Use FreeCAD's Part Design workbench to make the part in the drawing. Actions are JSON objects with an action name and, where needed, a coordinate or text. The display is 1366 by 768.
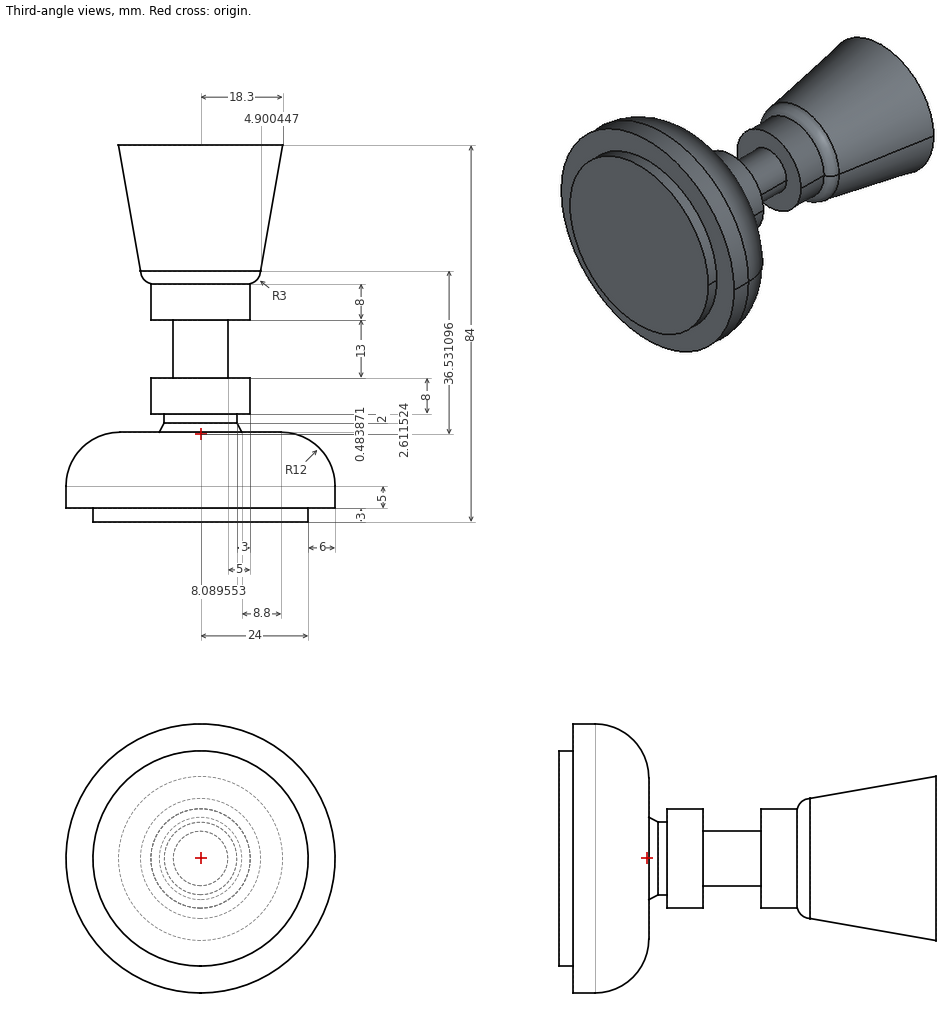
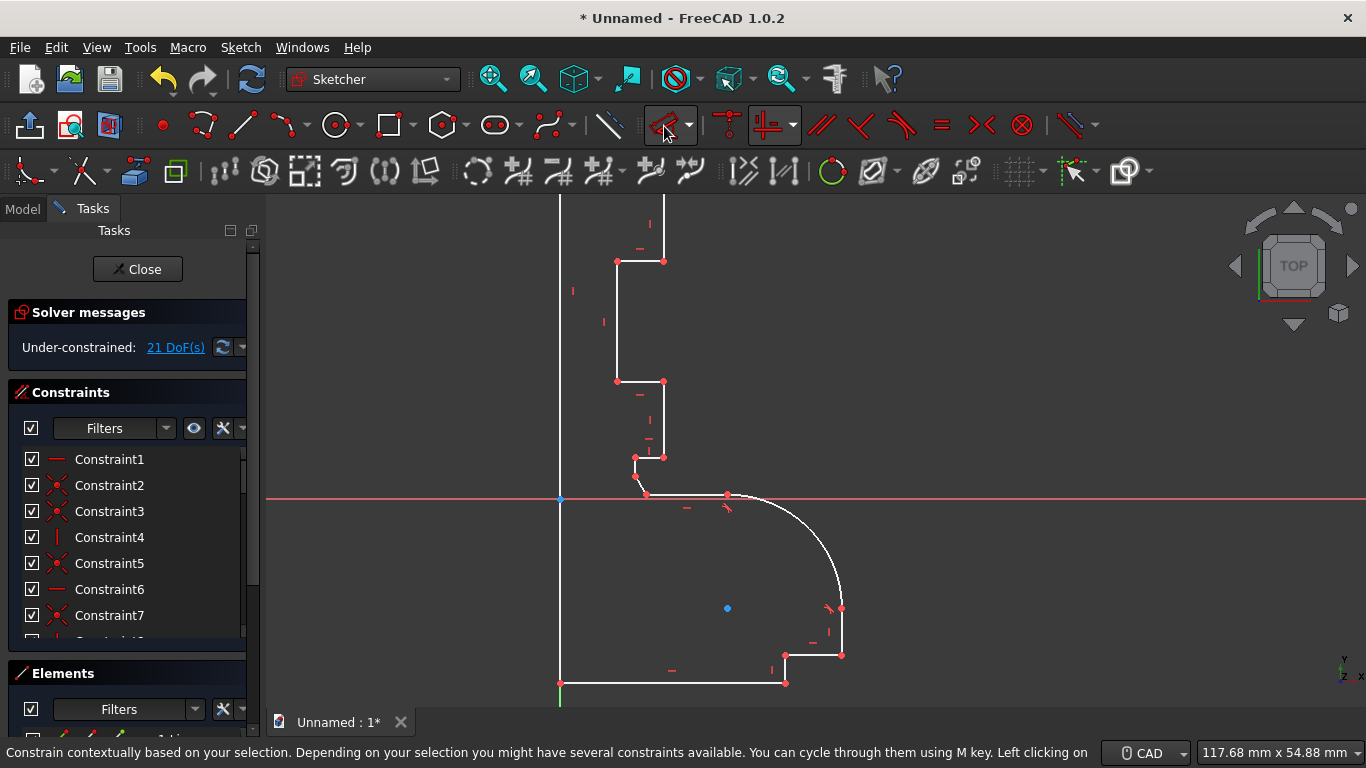
{"action": "scroll", "coordinate": [786, 582], "scroll_direction": "down", "scroll_amount": 4}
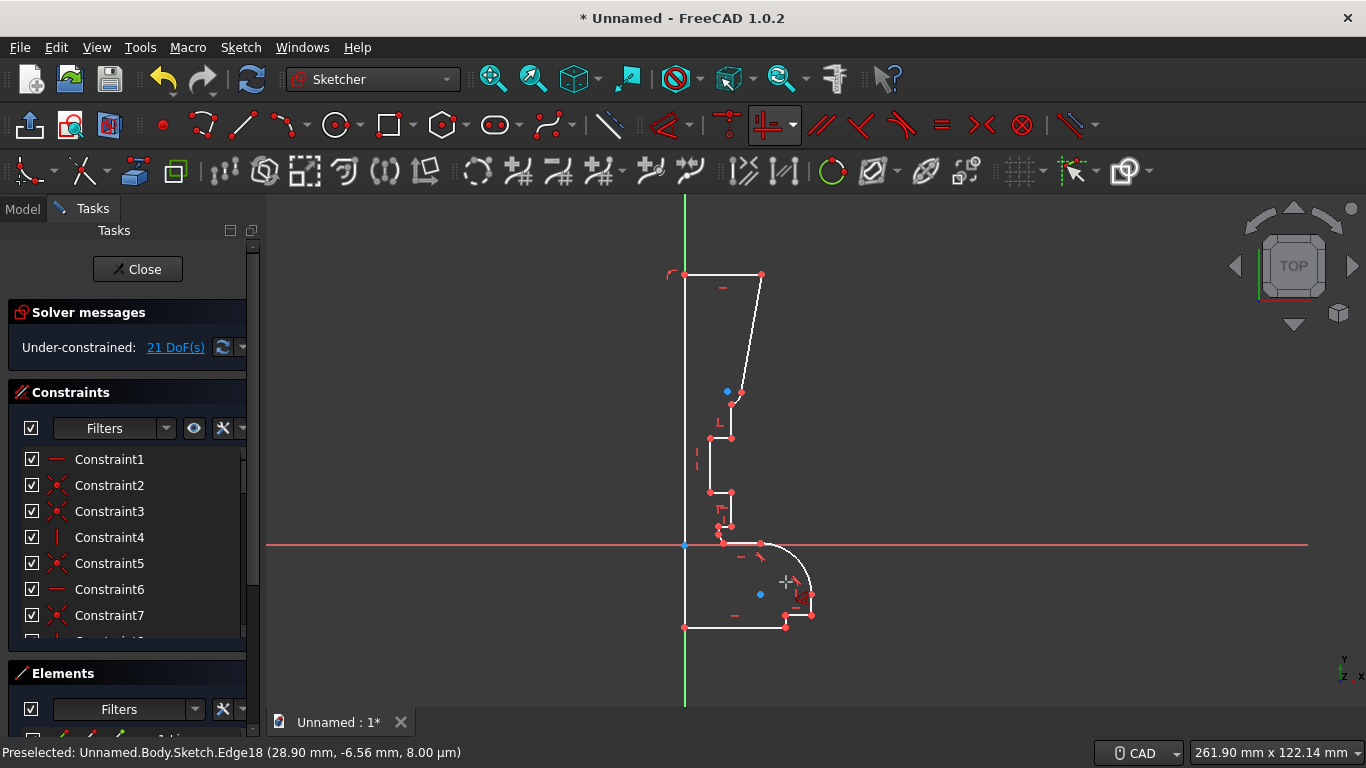
{"action": "scroll", "coordinate": [736, 402], "scroll_direction": "up", "scroll_amount": 6}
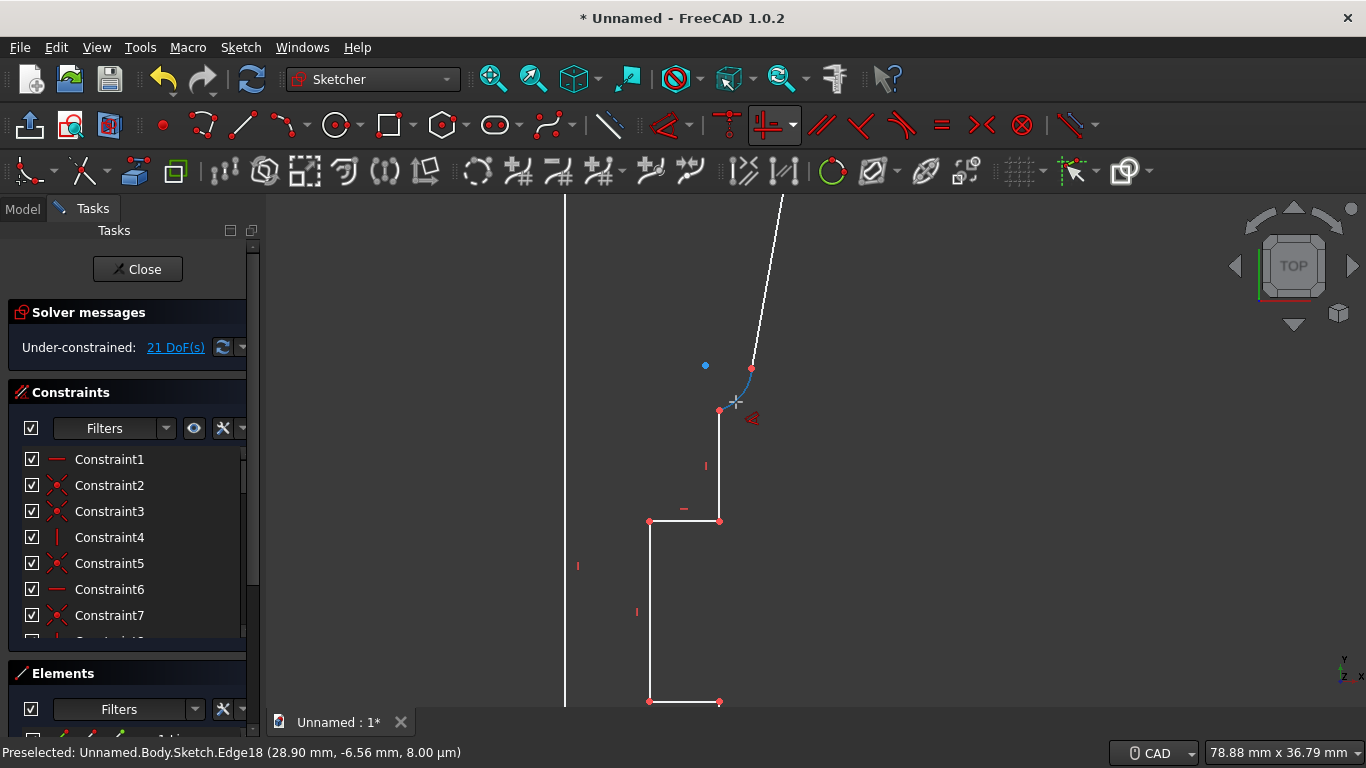
{"action": "left_click", "coordinate": [734, 402]}
{"action": "left_click", "coordinate": [754, 427]}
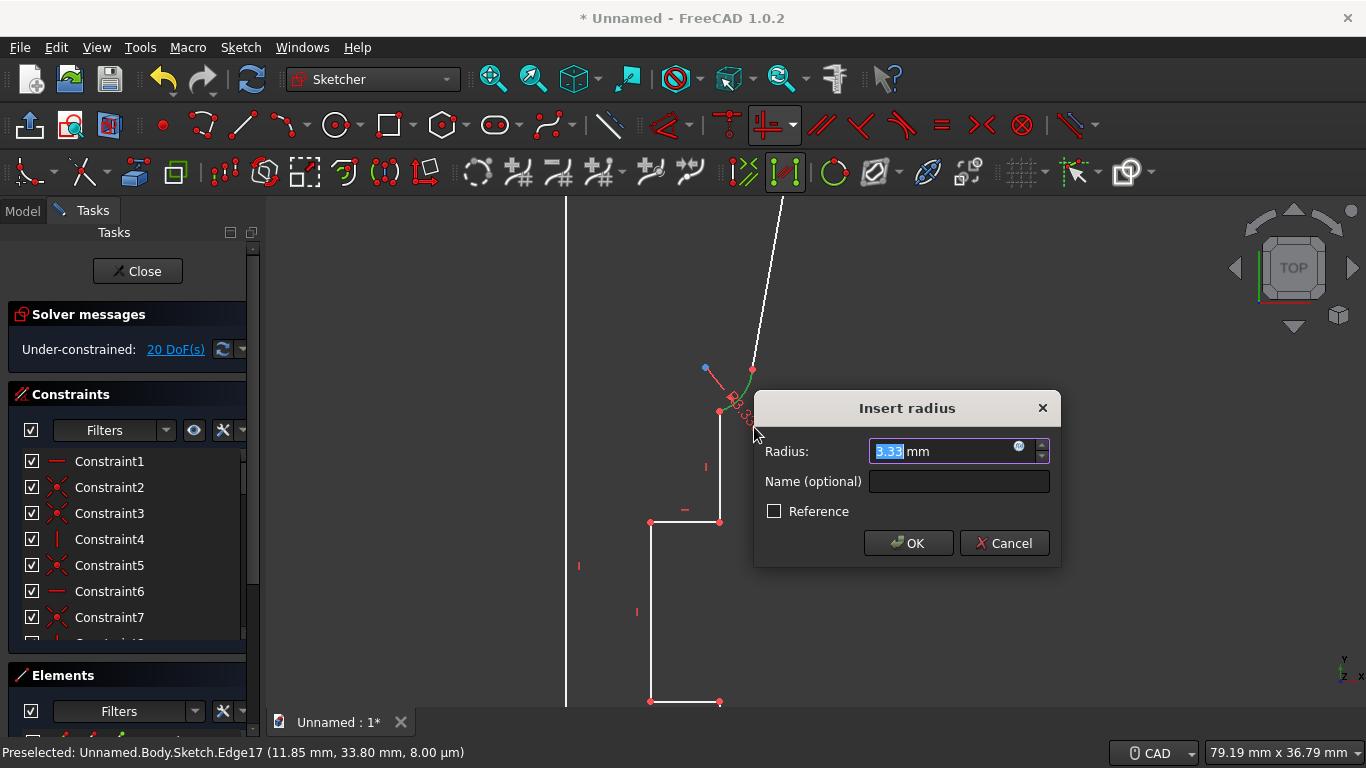
{"action": "type", "text": "3"}
{"action": "key", "text": "Return"}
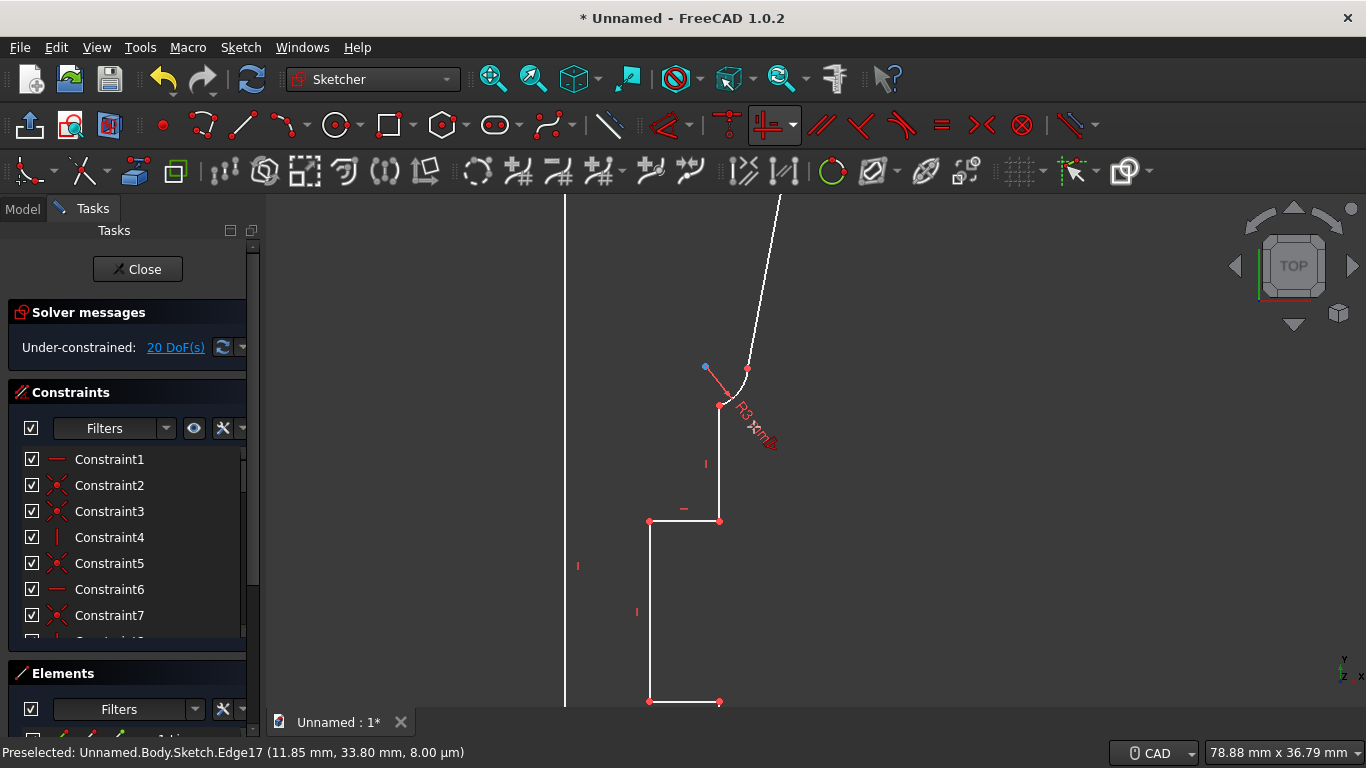
{"action": "scroll", "coordinate": [736, 402], "scroll_direction": "down", "scroll_amount": 6}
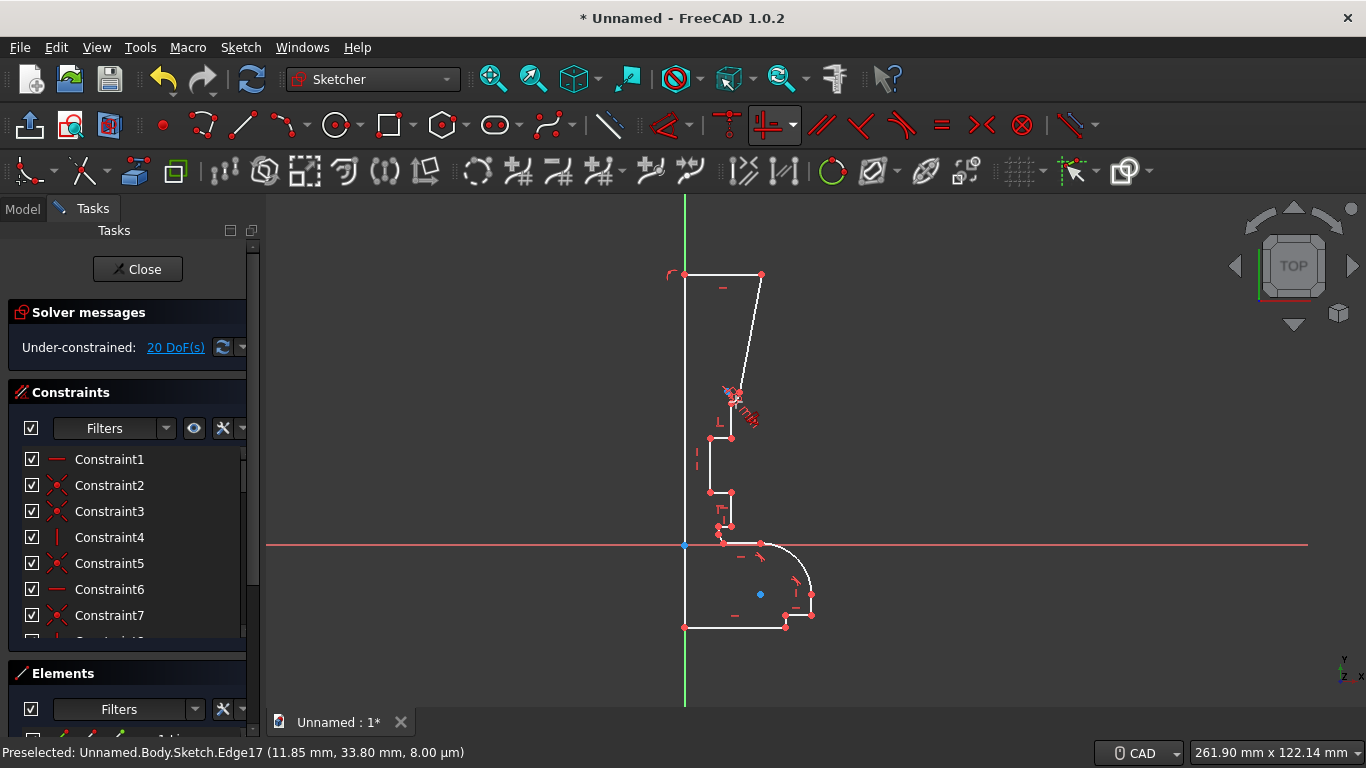
{"action": "left_click", "coordinate": [806, 571]}
{"action": "left_click", "coordinate": [844, 597]}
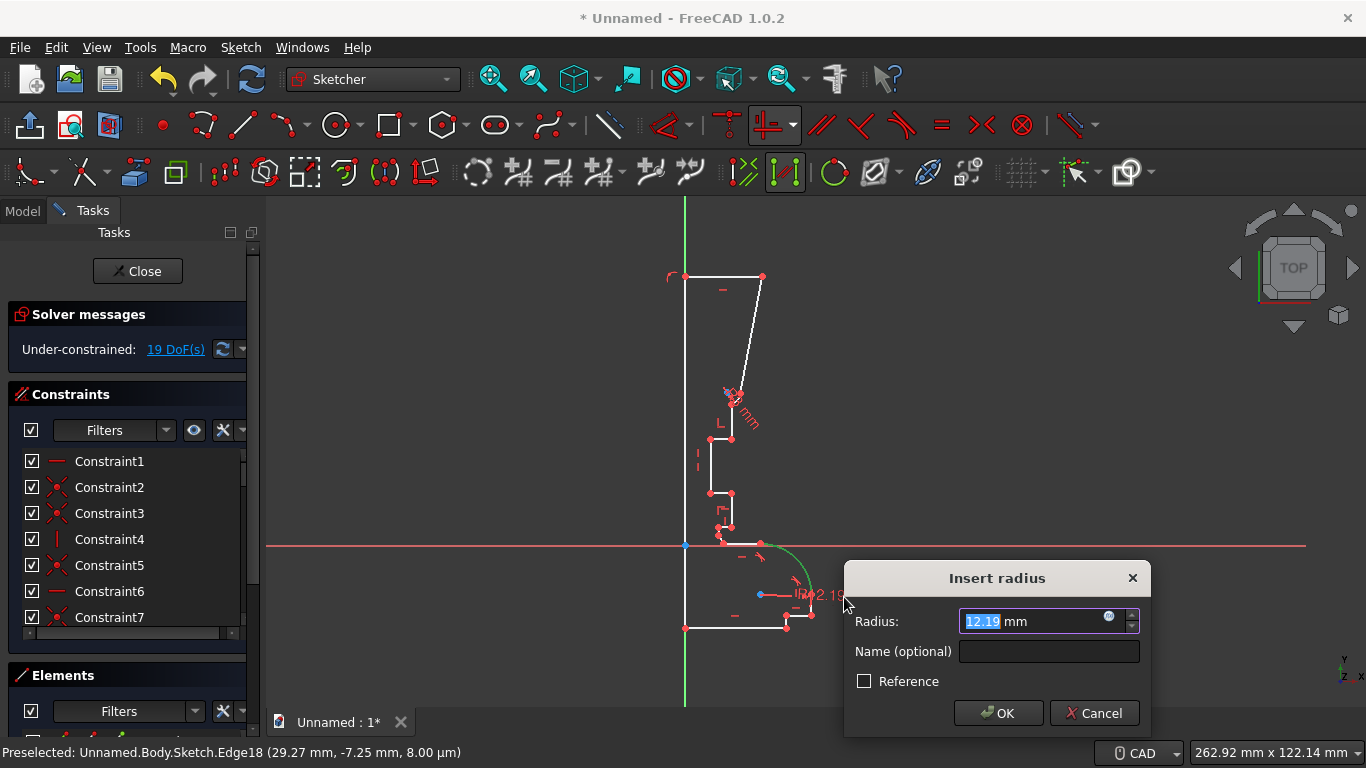
{"action": "type", "text": "12"}
{"action": "key", "text": "Return"}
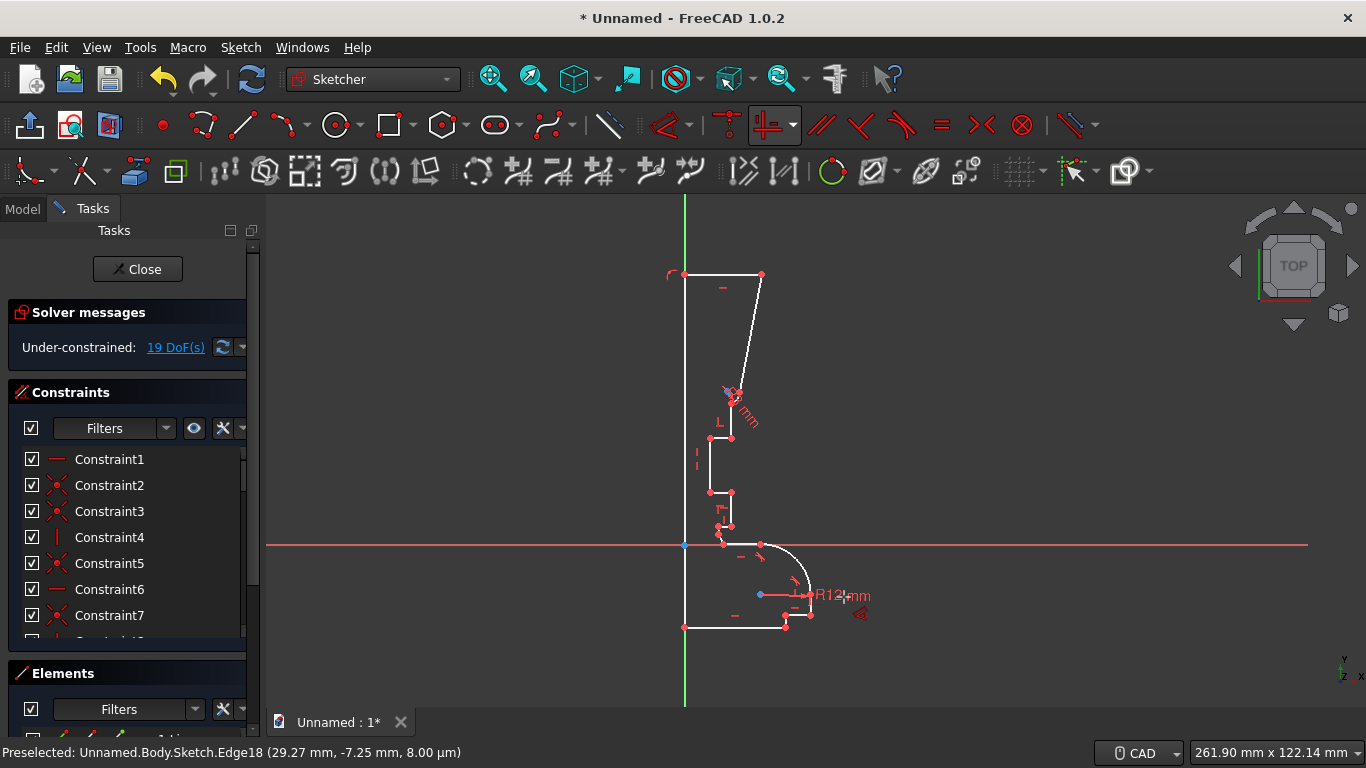
{"action": "scroll", "coordinate": [719, 531], "scroll_direction": "up", "scroll_amount": 8}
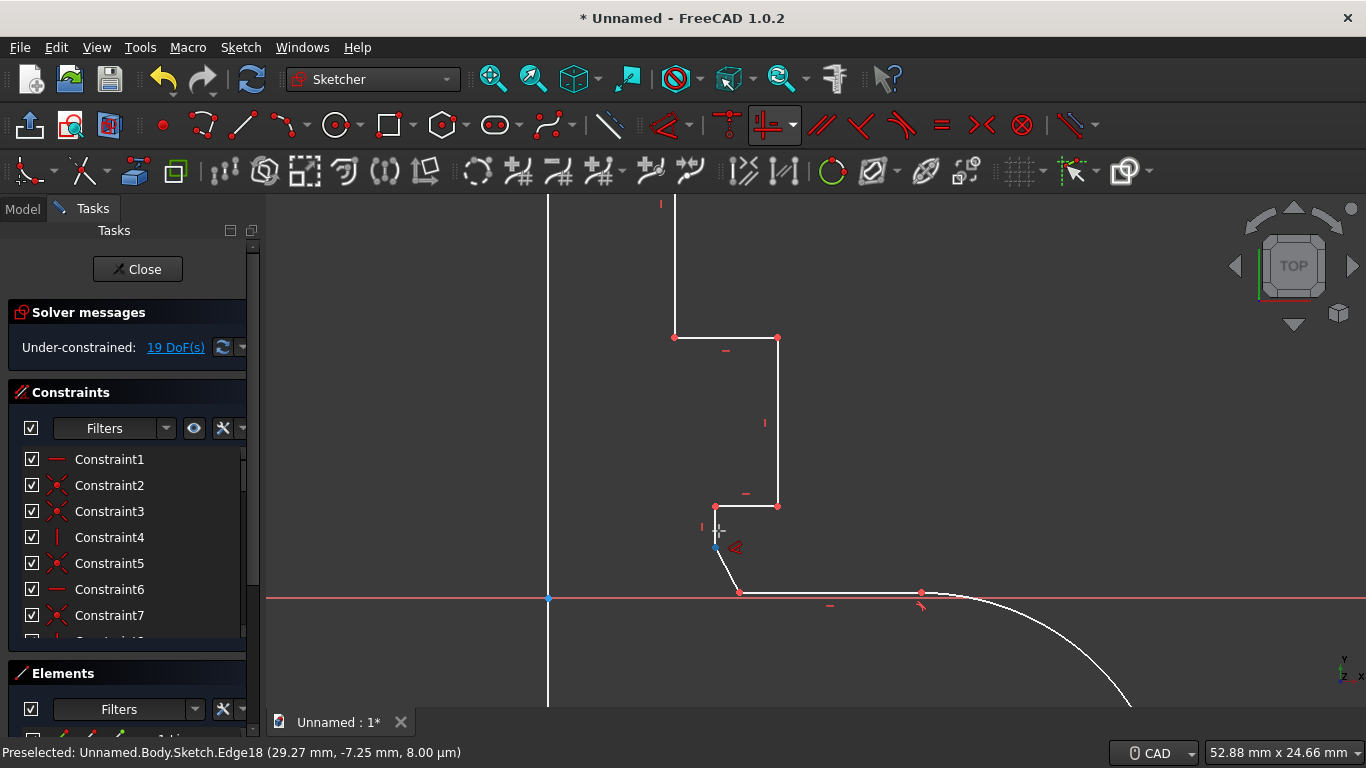
{"action": "left_click", "coordinate": [715, 527]}
{"action": "left_click", "coordinate": [681, 527]}